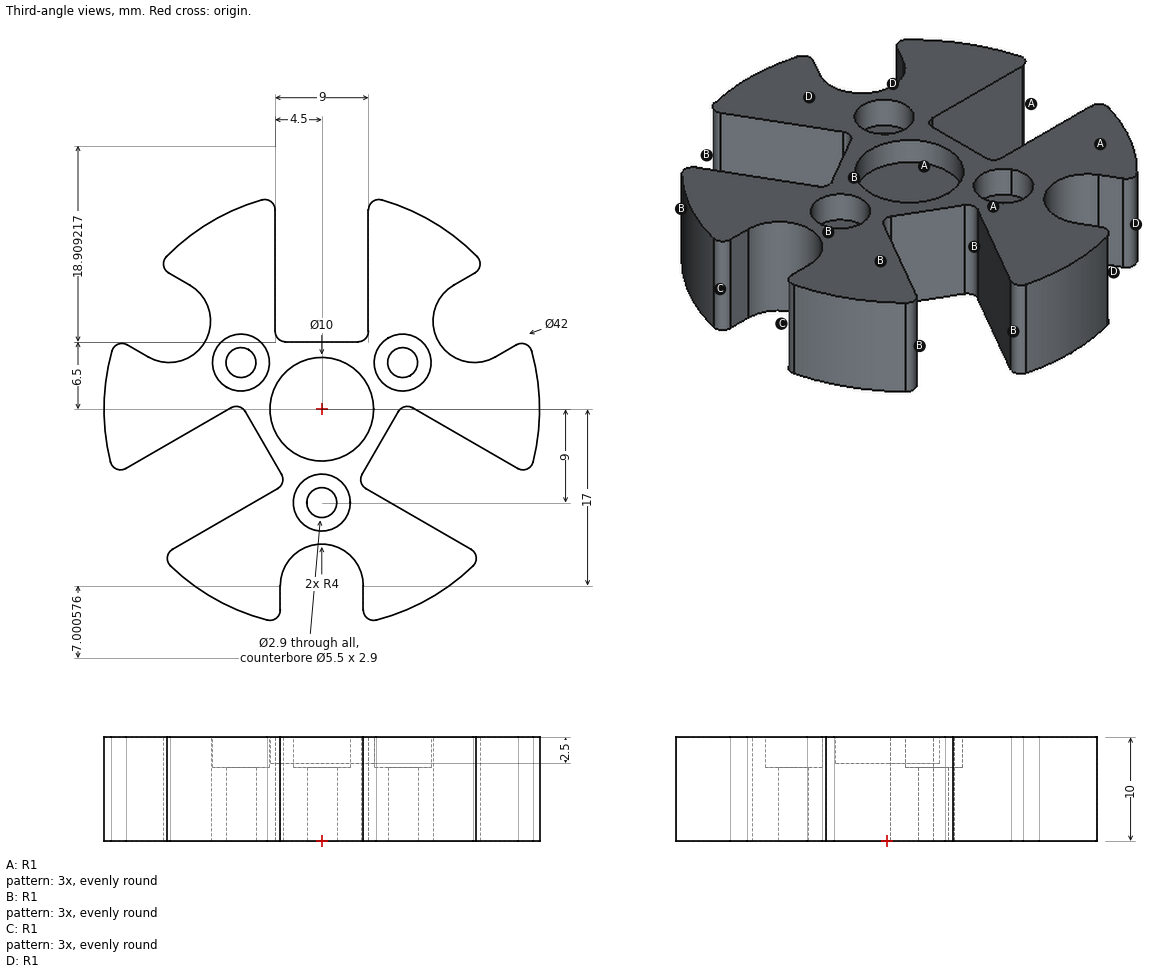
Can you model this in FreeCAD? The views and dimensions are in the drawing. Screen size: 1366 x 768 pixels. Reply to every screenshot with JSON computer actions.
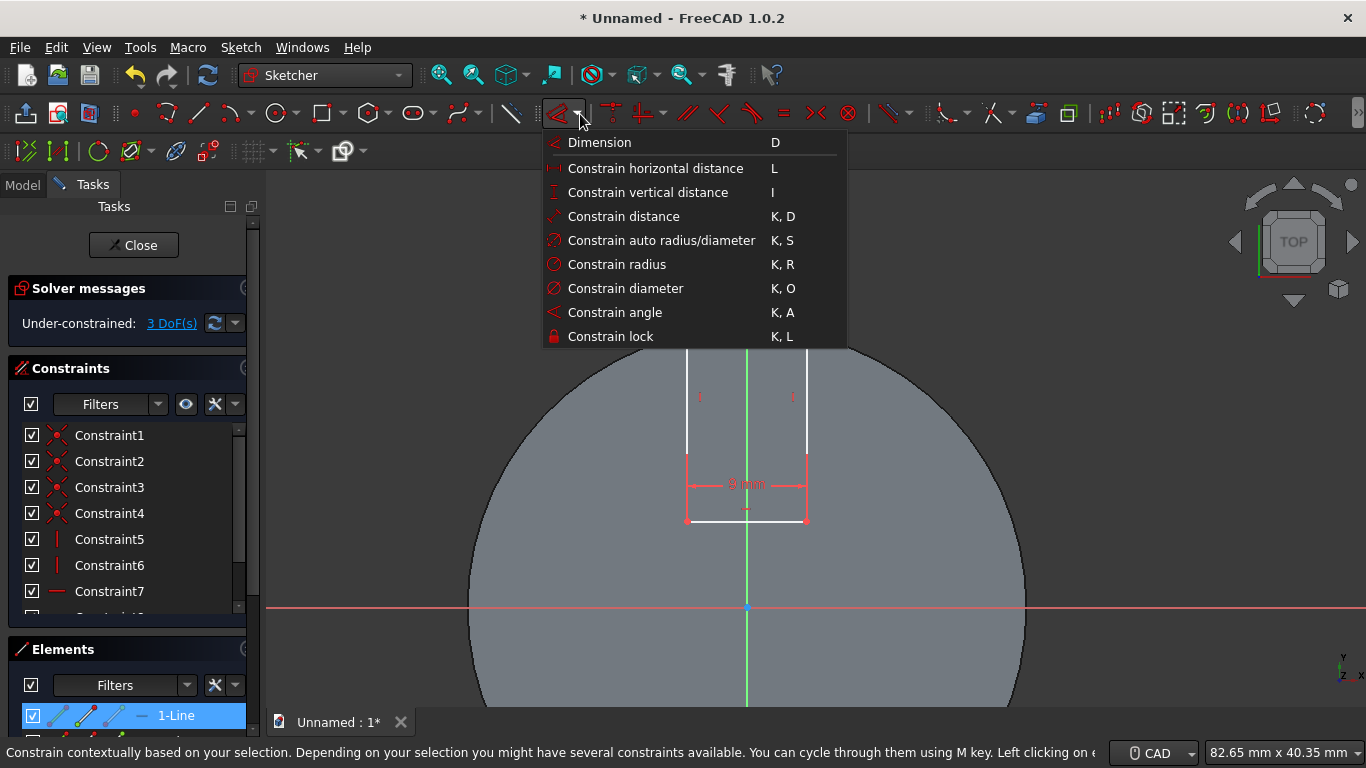
{"action": "left_click", "coordinate": [695, 168]}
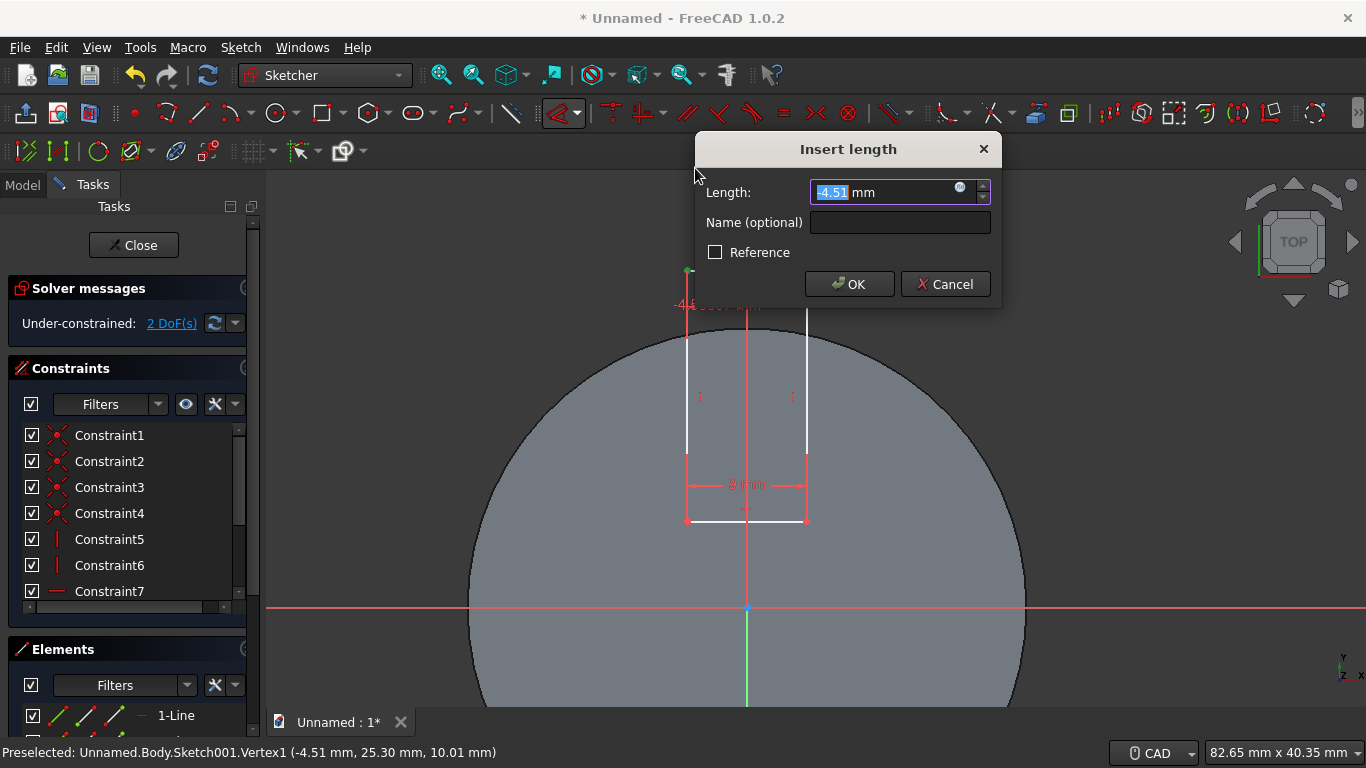
{"action": "type", "text": "-4.5"}
{"action": "key", "text": "Return"}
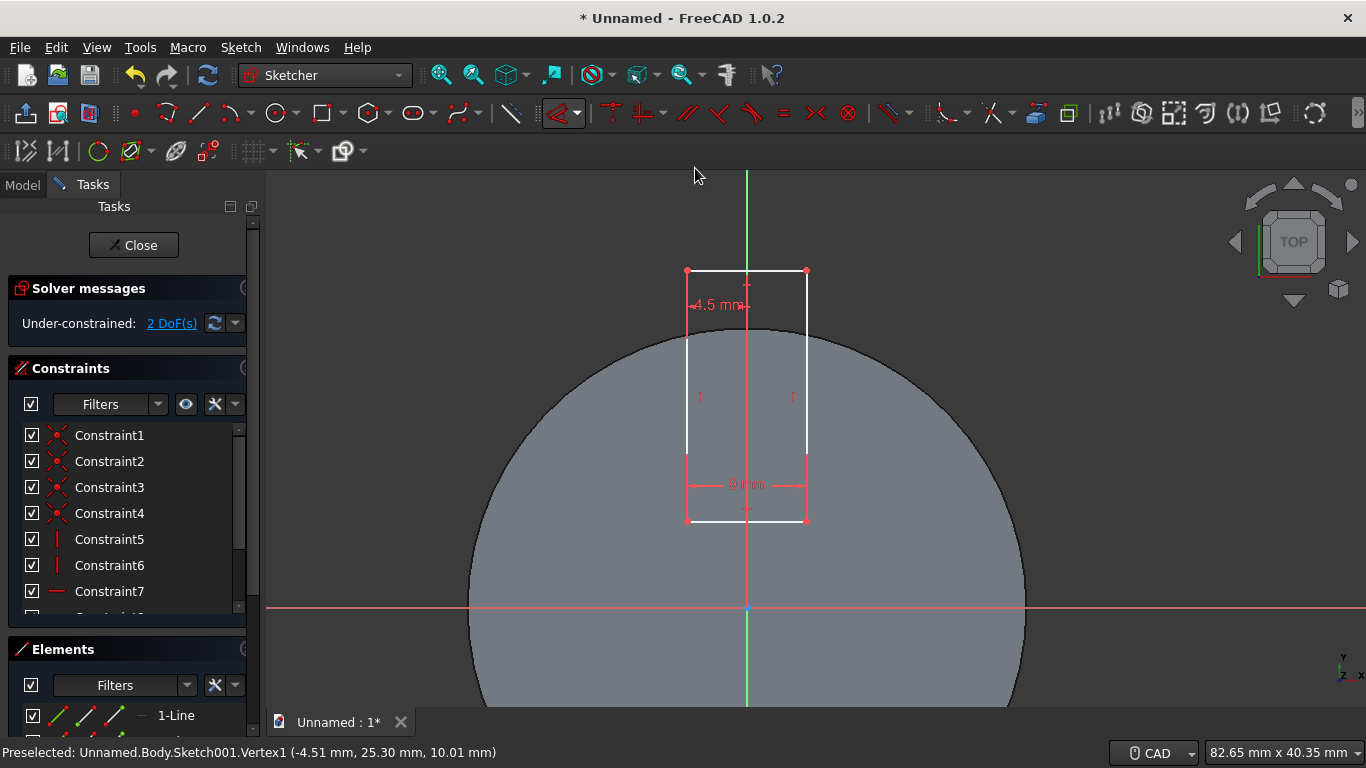
{"action": "left_click", "coordinate": [687, 522]}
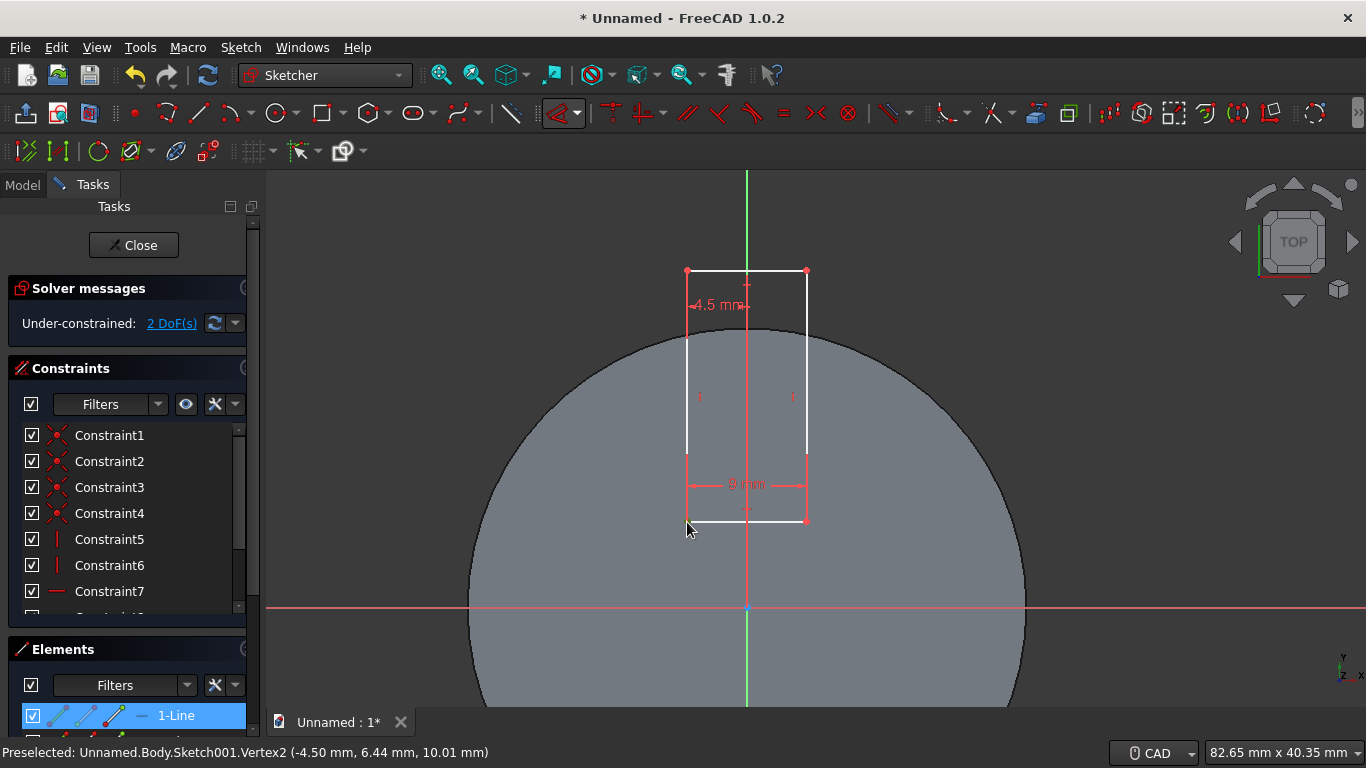
{"action": "left_click", "coordinate": [580, 114]}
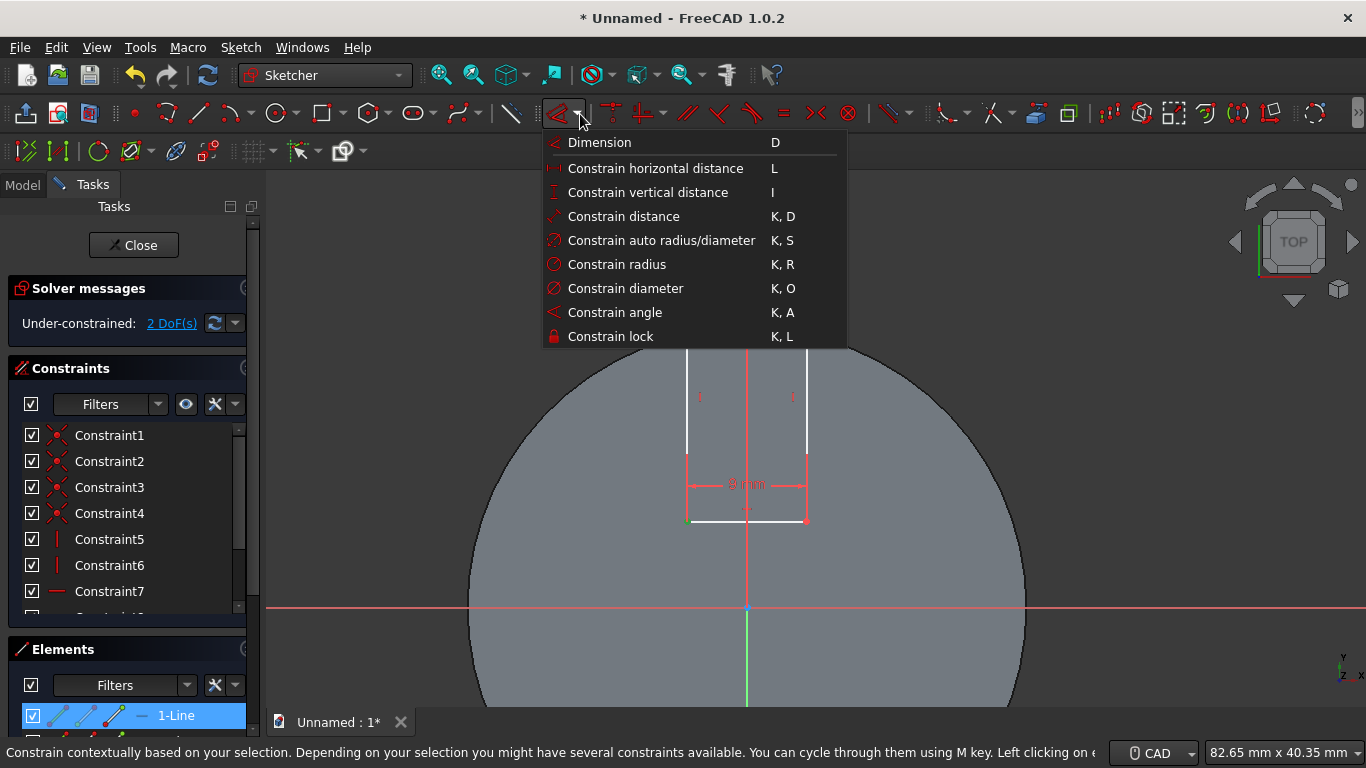
{"action": "left_click", "coordinate": [695, 192]}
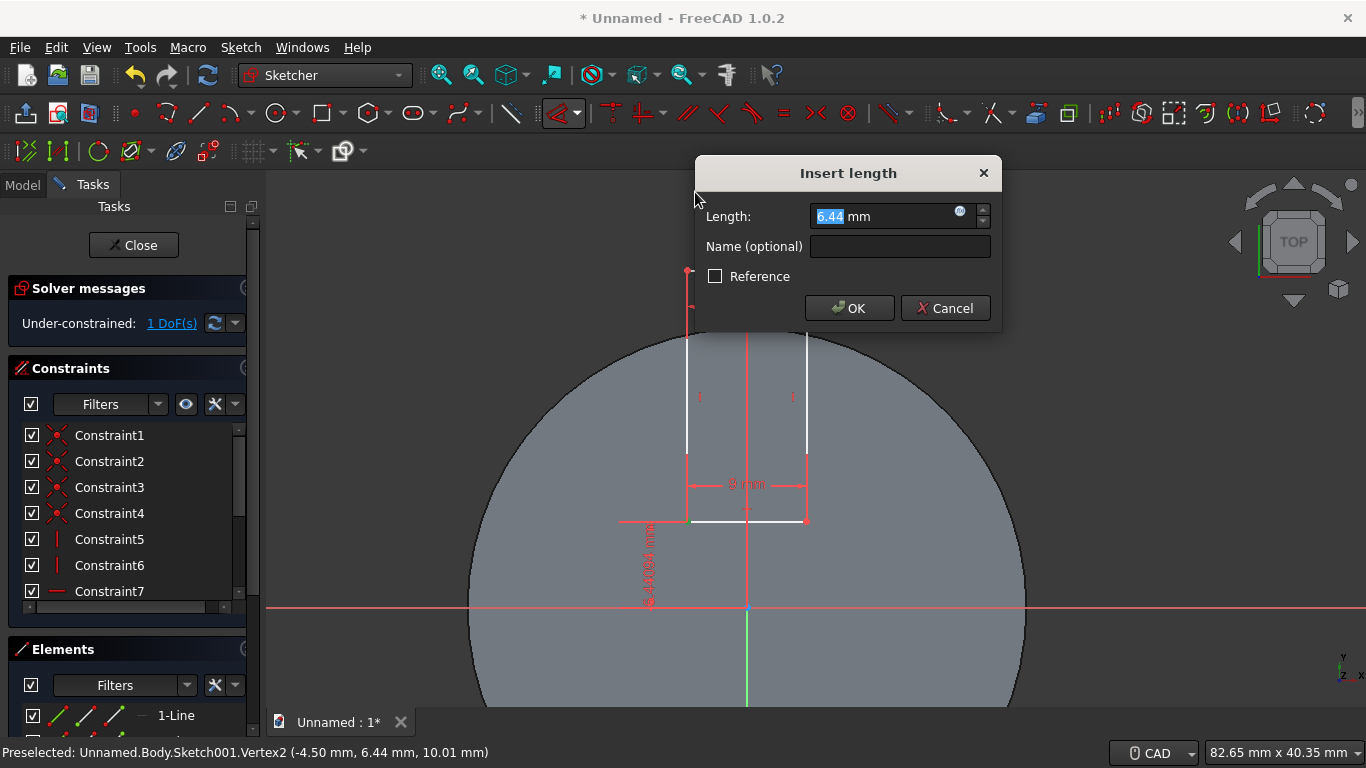
{"action": "type", "text": "6.5"}
{"action": "key", "text": "Return"}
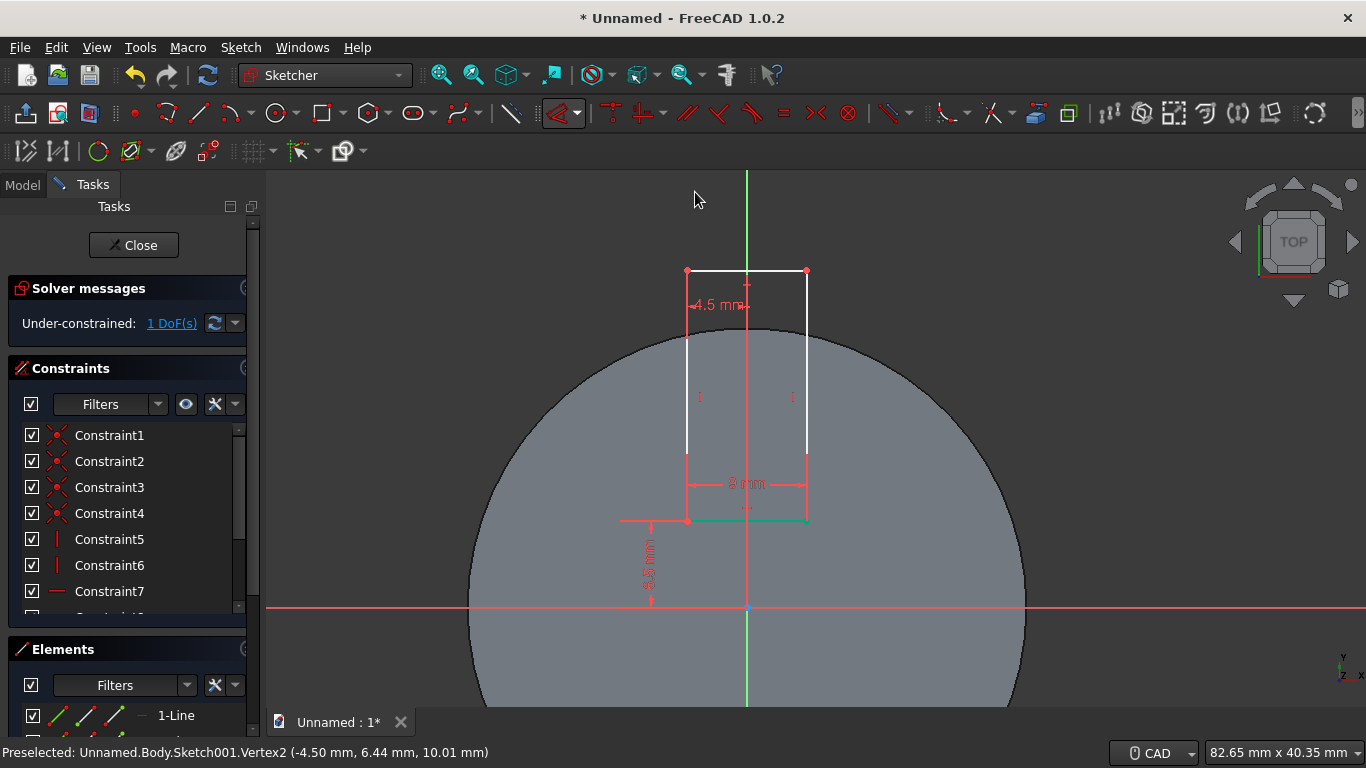
{"action": "left_click", "coordinate": [687, 346]}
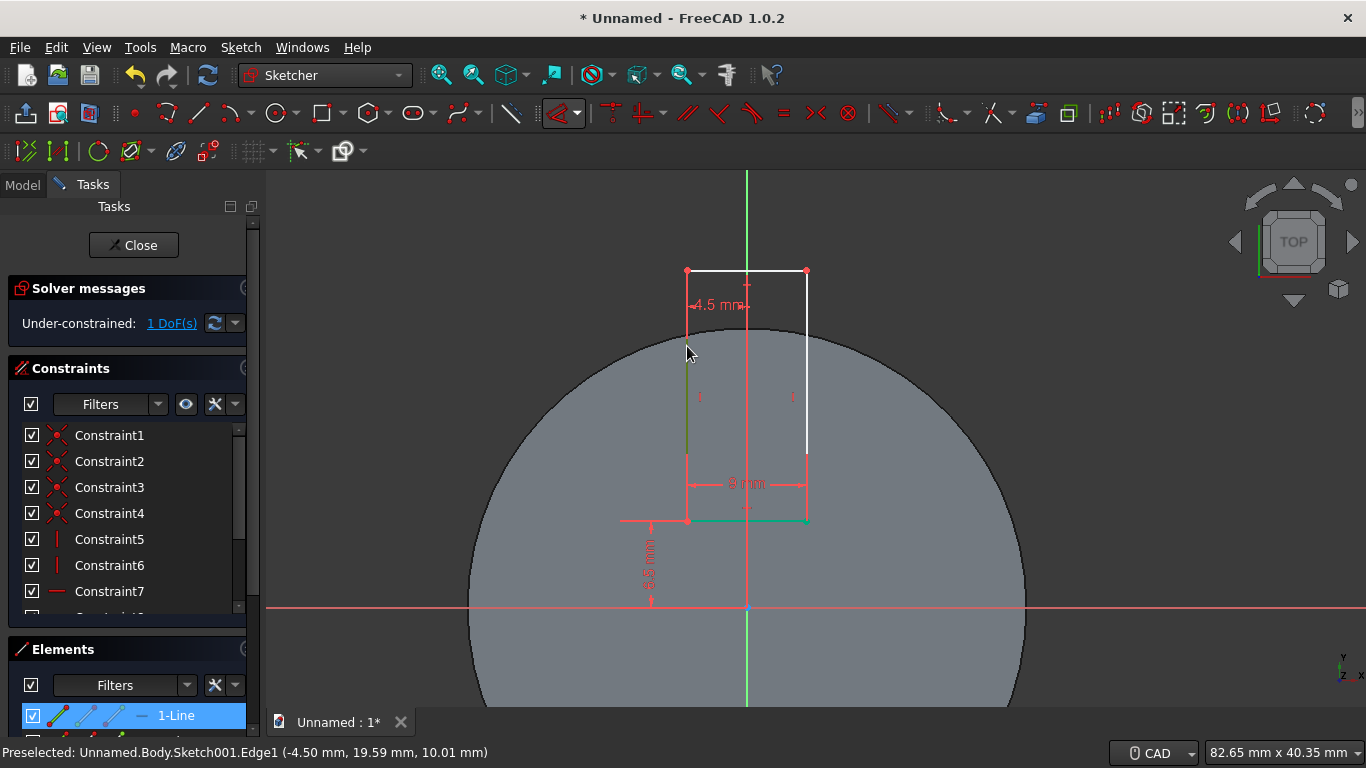
{"action": "left_click", "coordinate": [580, 114]}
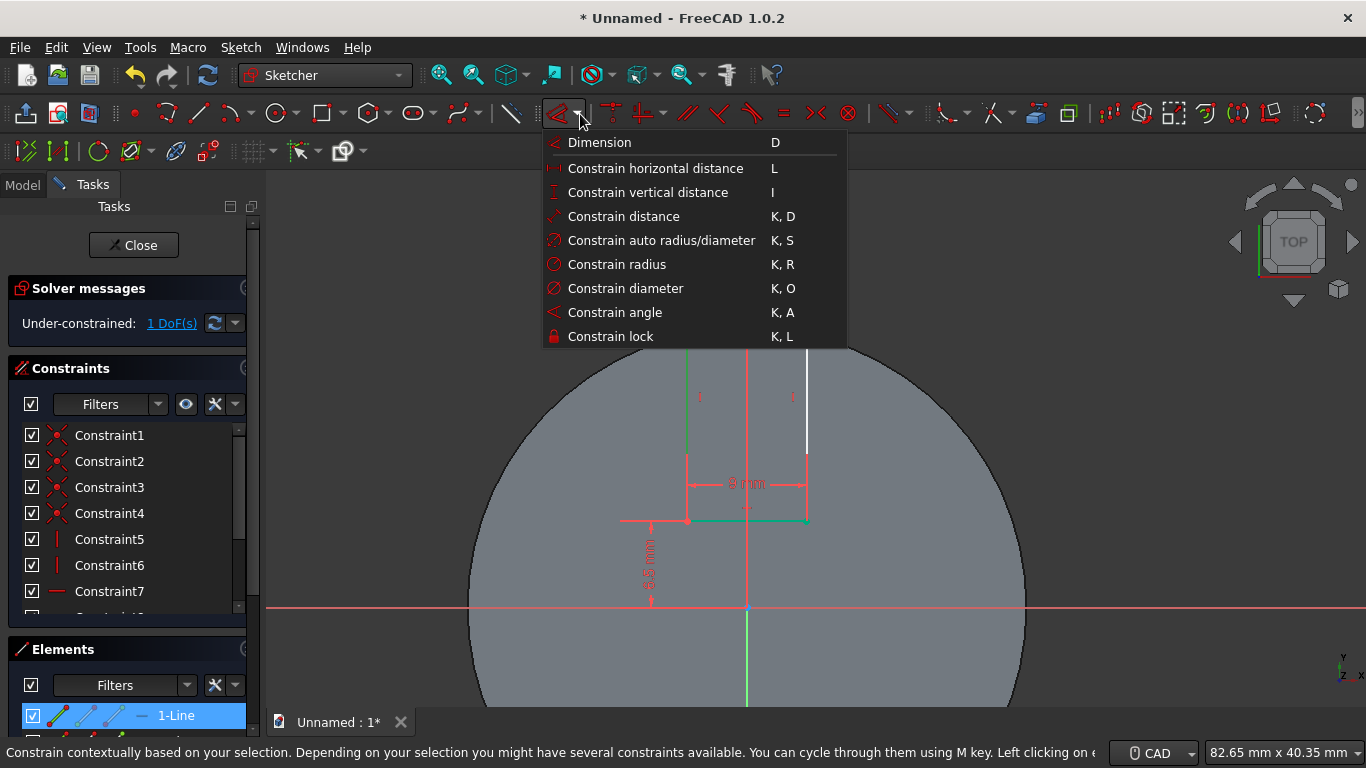
{"action": "left_click", "coordinate": [695, 192]}